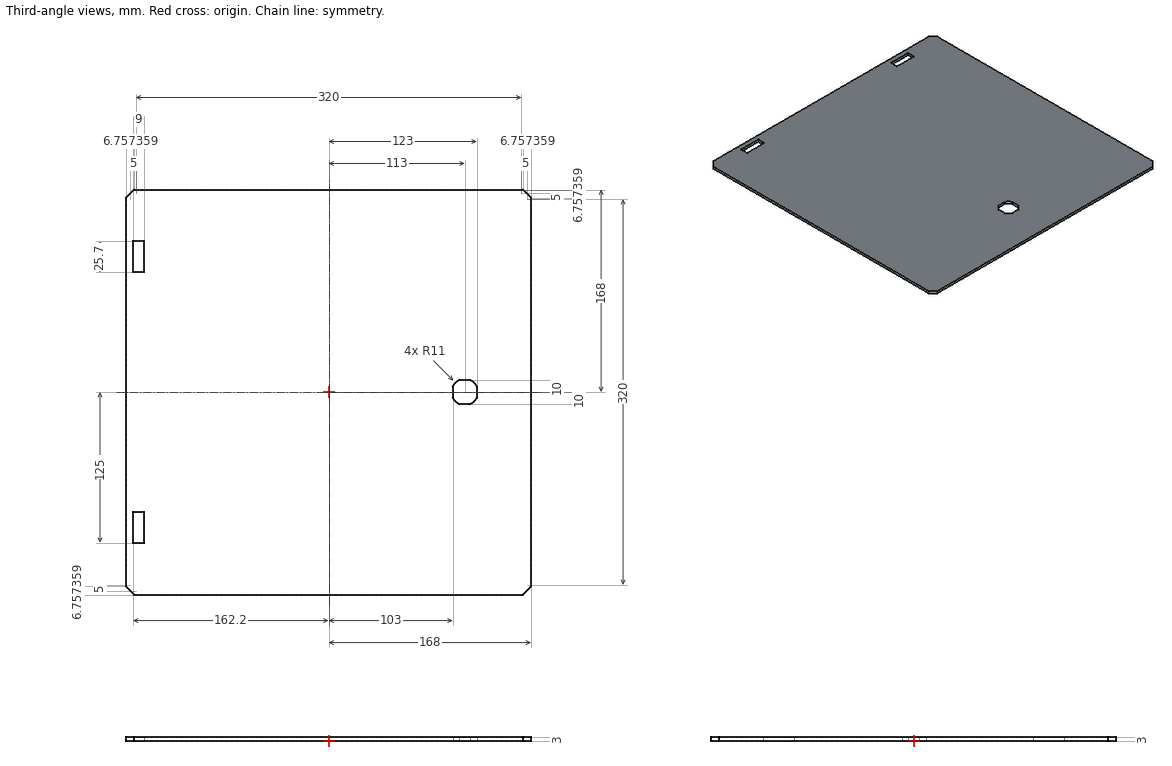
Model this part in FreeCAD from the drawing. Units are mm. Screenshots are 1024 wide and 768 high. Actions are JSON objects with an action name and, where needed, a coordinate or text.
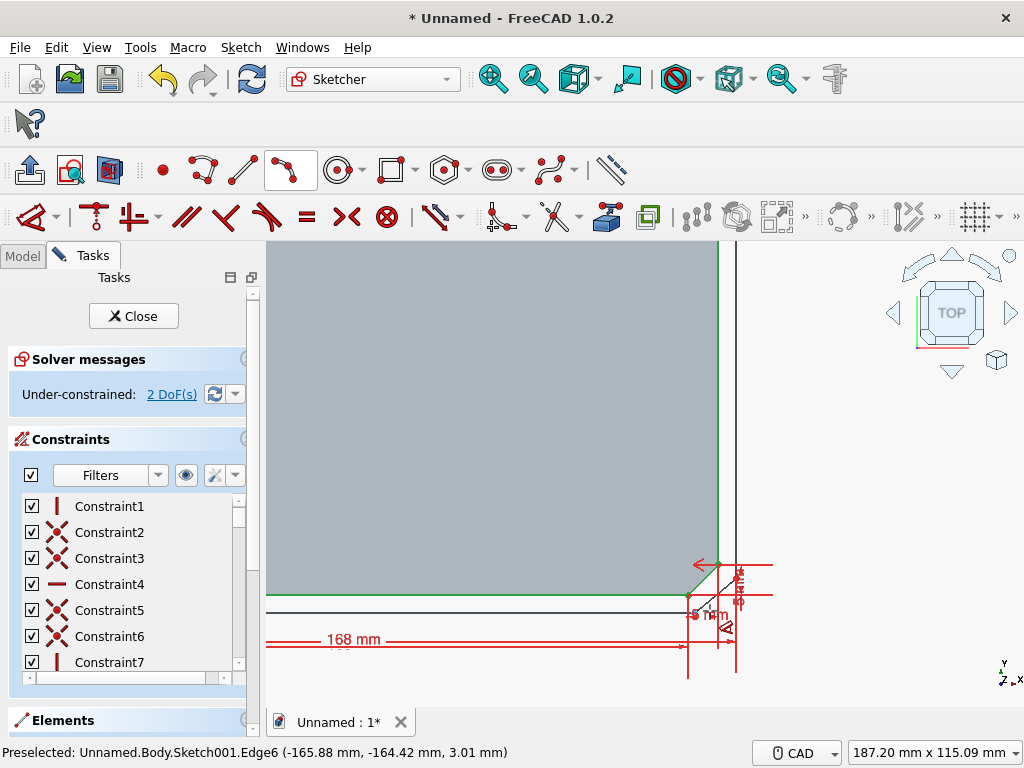
{"action": "left_click", "coordinate": [707, 603]}
{"action": "left_click", "coordinate": [716, 647]}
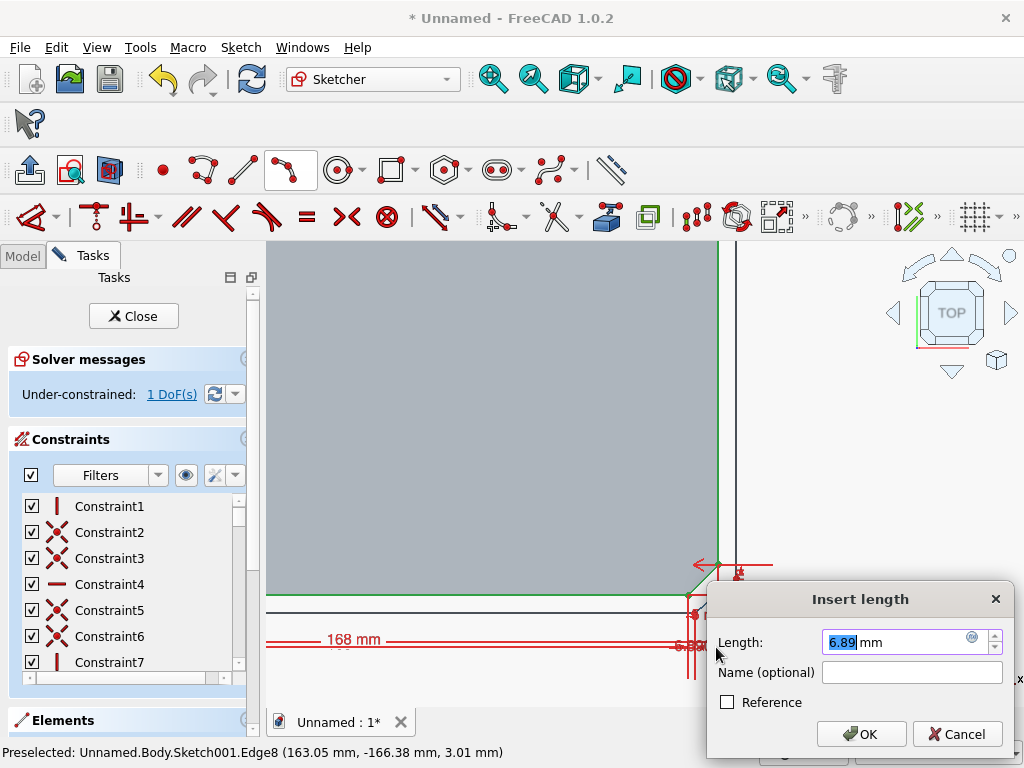
{"action": "type", "text": "6.757359"}
{"action": "key", "text": "Return"}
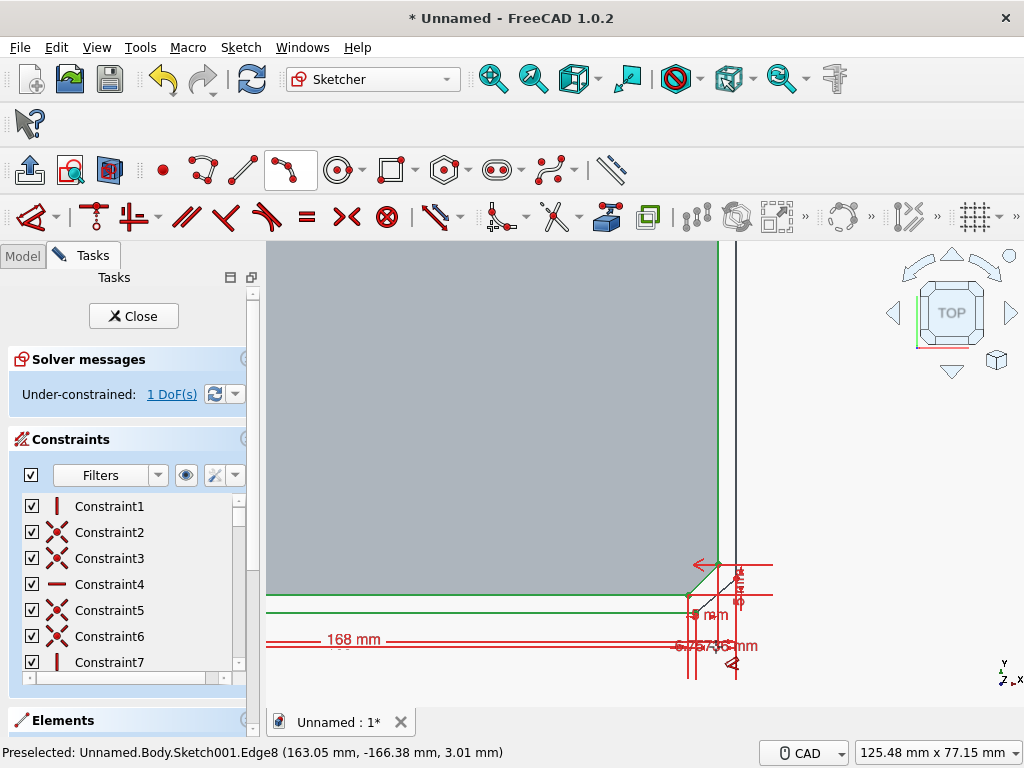
{"action": "left_click", "coordinate": [708, 603]}
{"action": "left_click", "coordinate": [794, 608]}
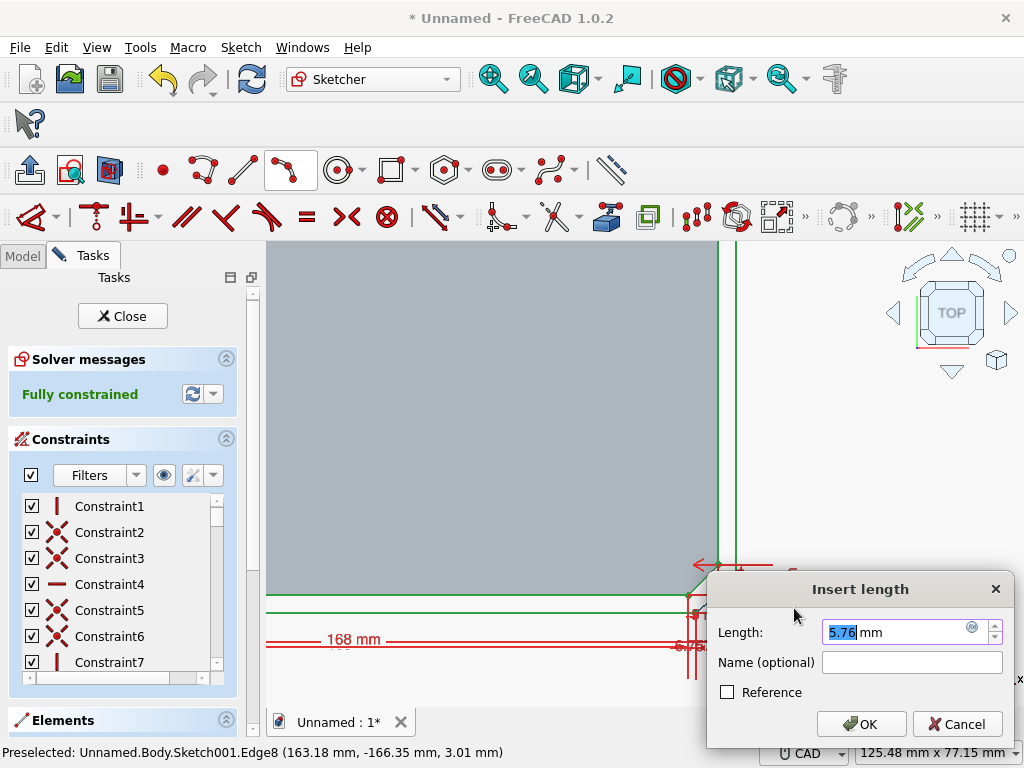
{"action": "type", "text": "6.757359"}
{"action": "key", "text": "Return"}
{"action": "key", "text": "Escape"}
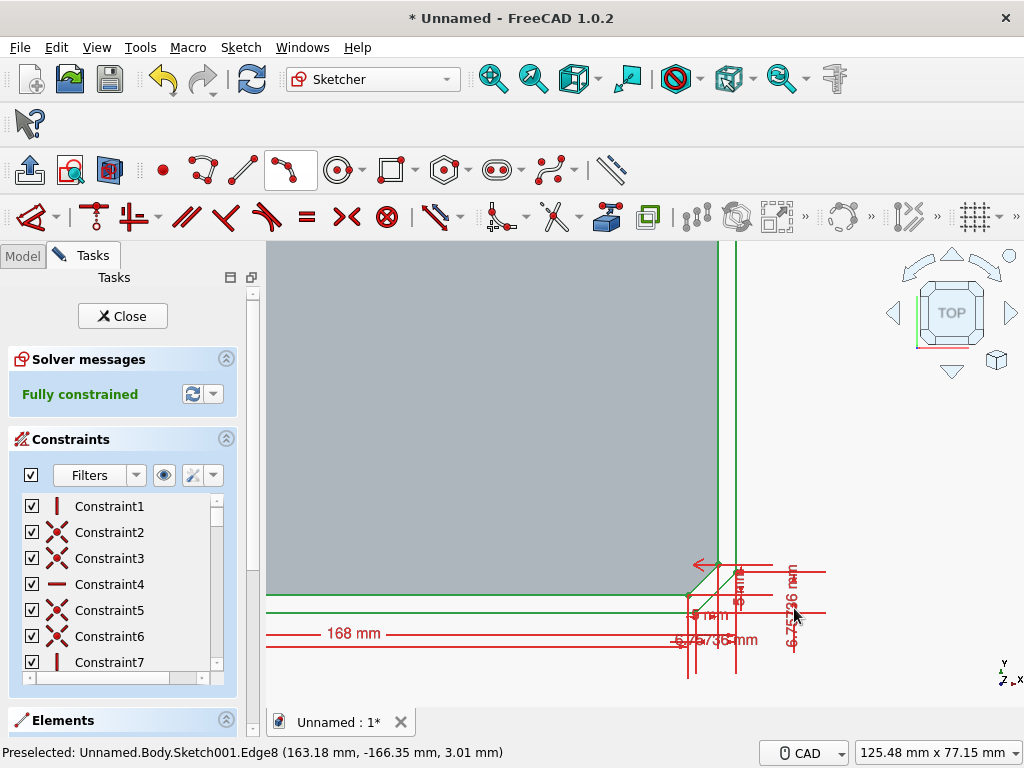
{"action": "left_click", "coordinate": [123, 316]}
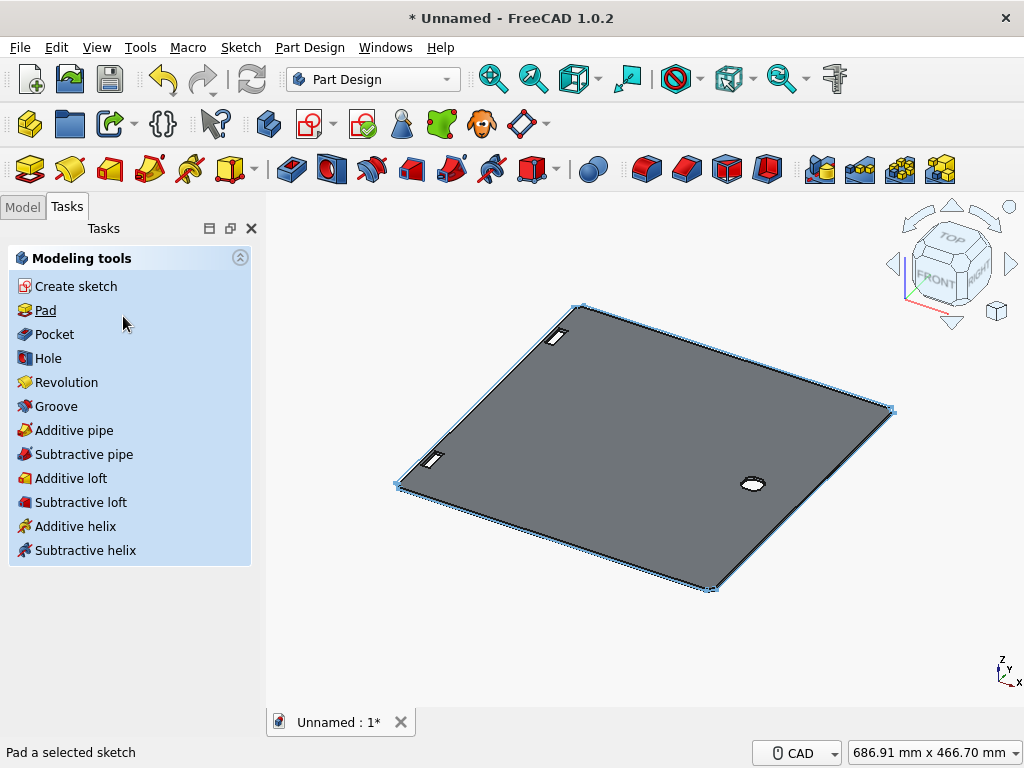
{"action": "left_click", "coordinate": [30, 170]}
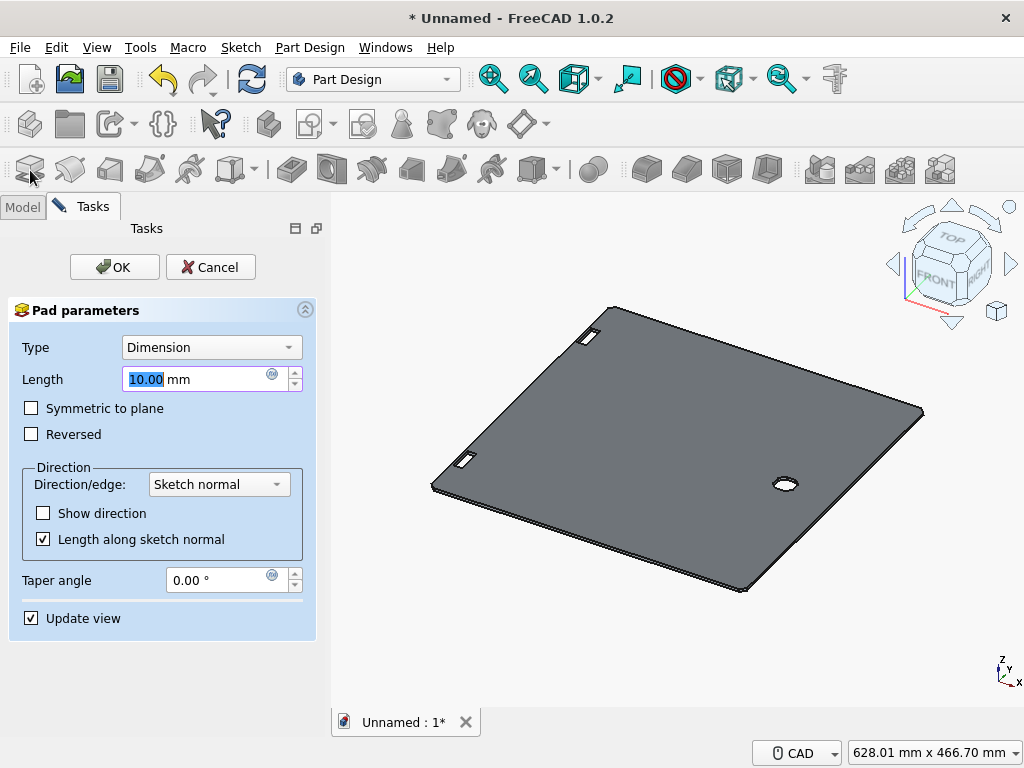
{"action": "type", "text": "3"}
{"action": "key", "text": "Tab"}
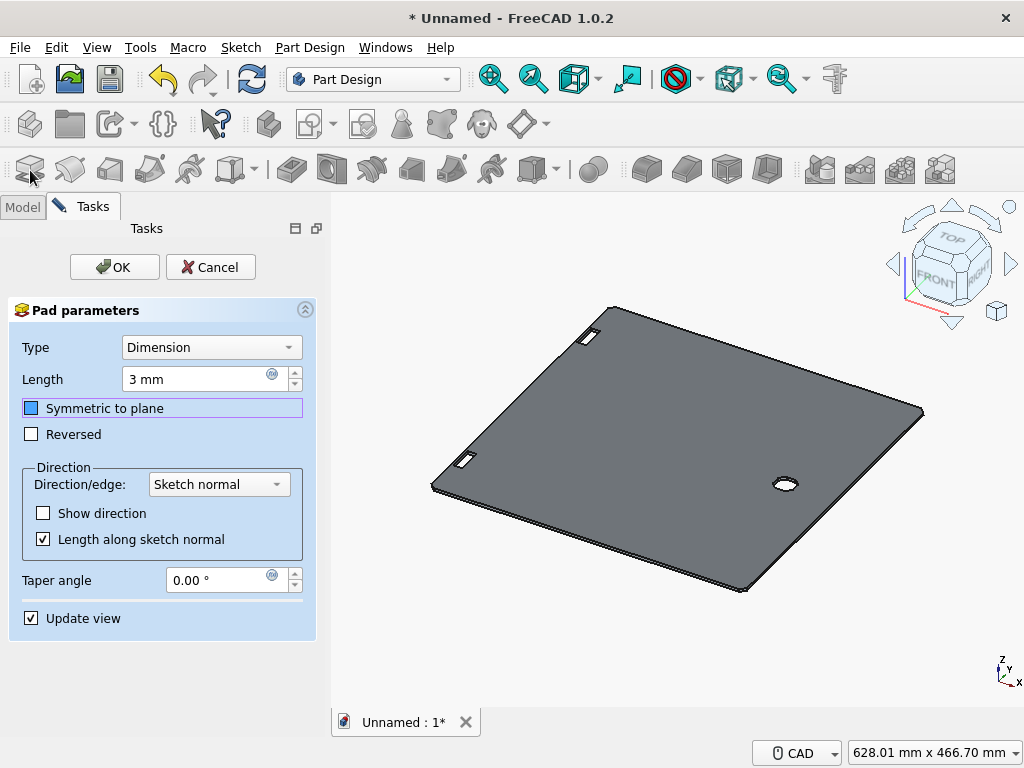
{"action": "left_click", "coordinate": [30, 434]}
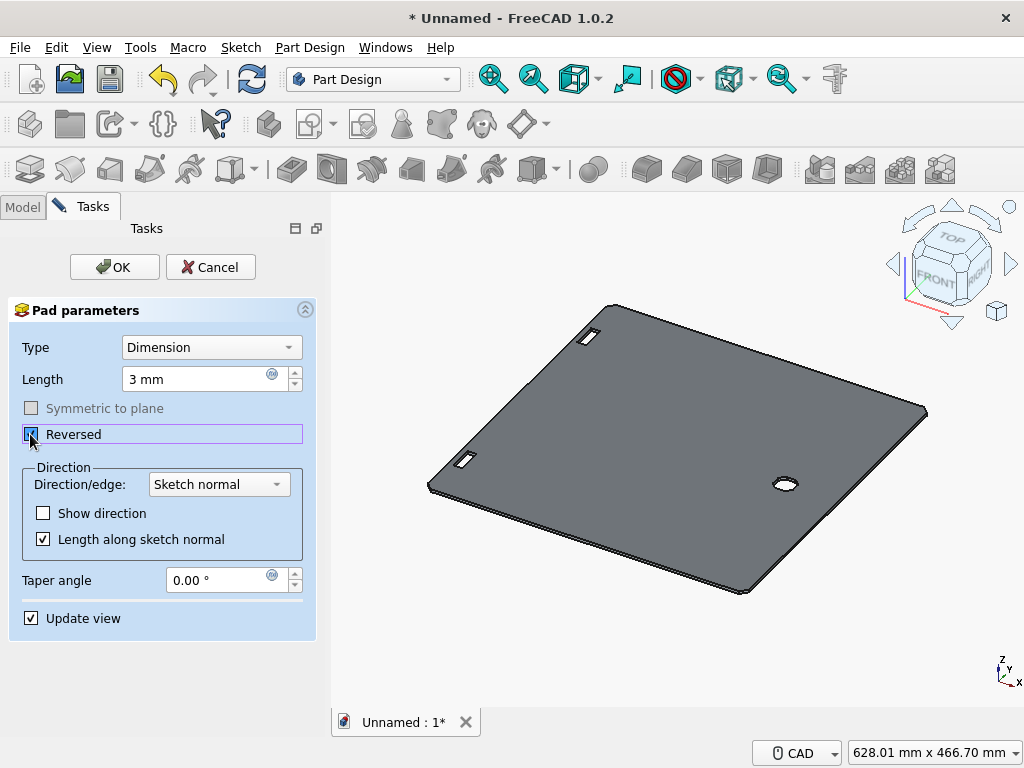
{"action": "left_click", "coordinate": [115, 267]}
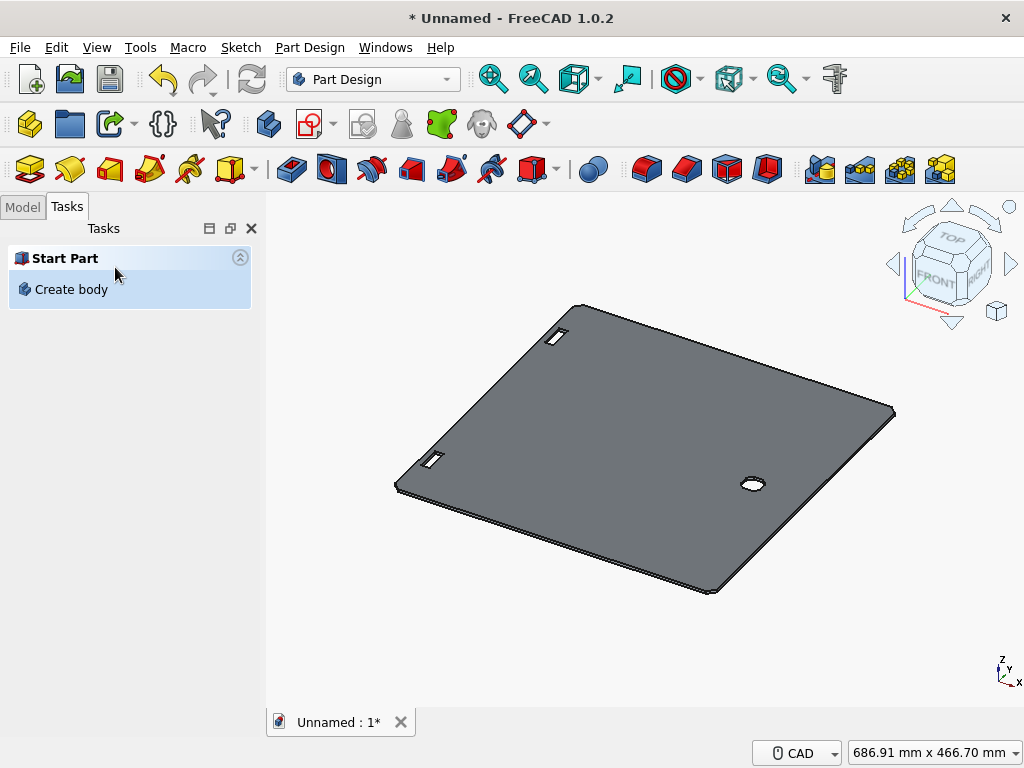
{"action": "key", "text": "0"}